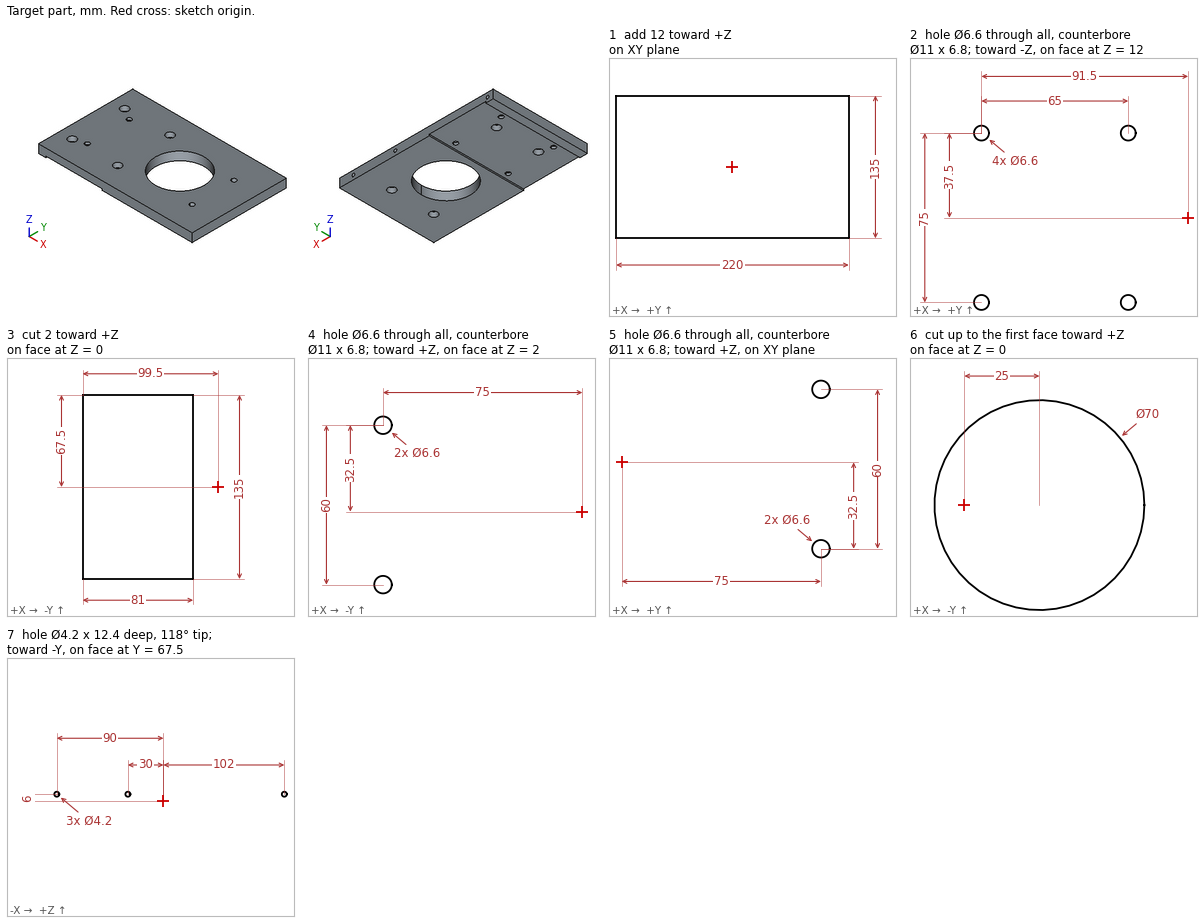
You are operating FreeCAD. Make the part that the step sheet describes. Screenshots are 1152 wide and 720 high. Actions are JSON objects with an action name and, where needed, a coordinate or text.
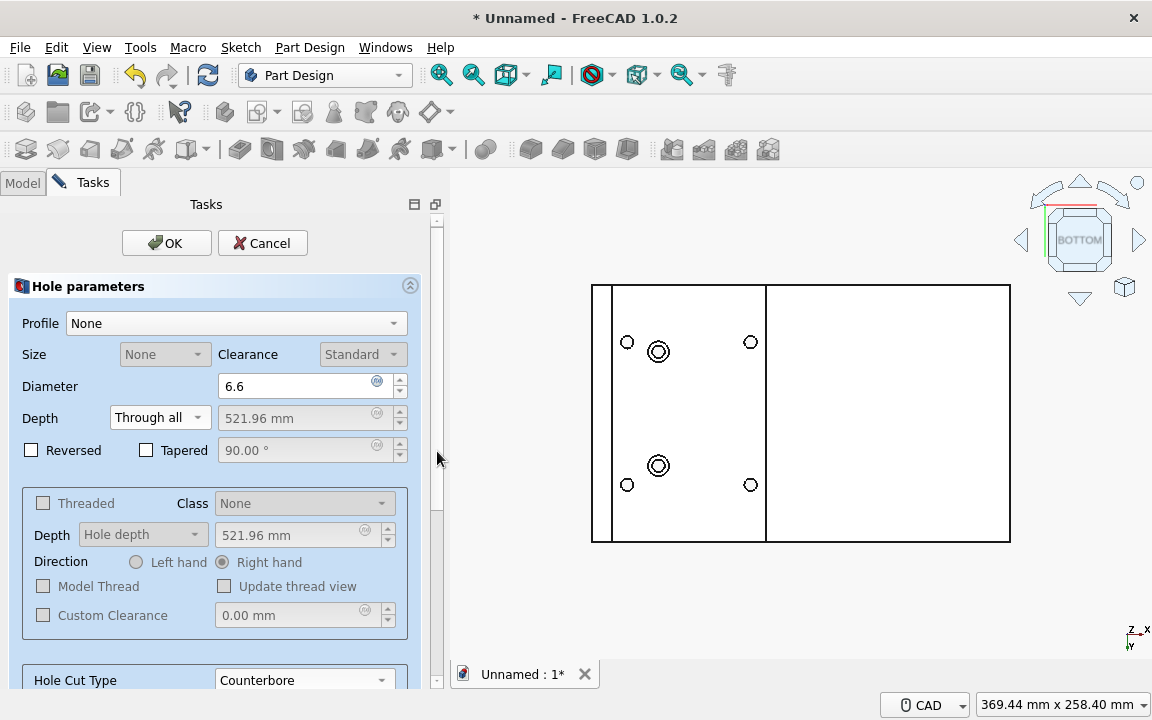
{"action": "left_click", "coordinate": [167, 243]}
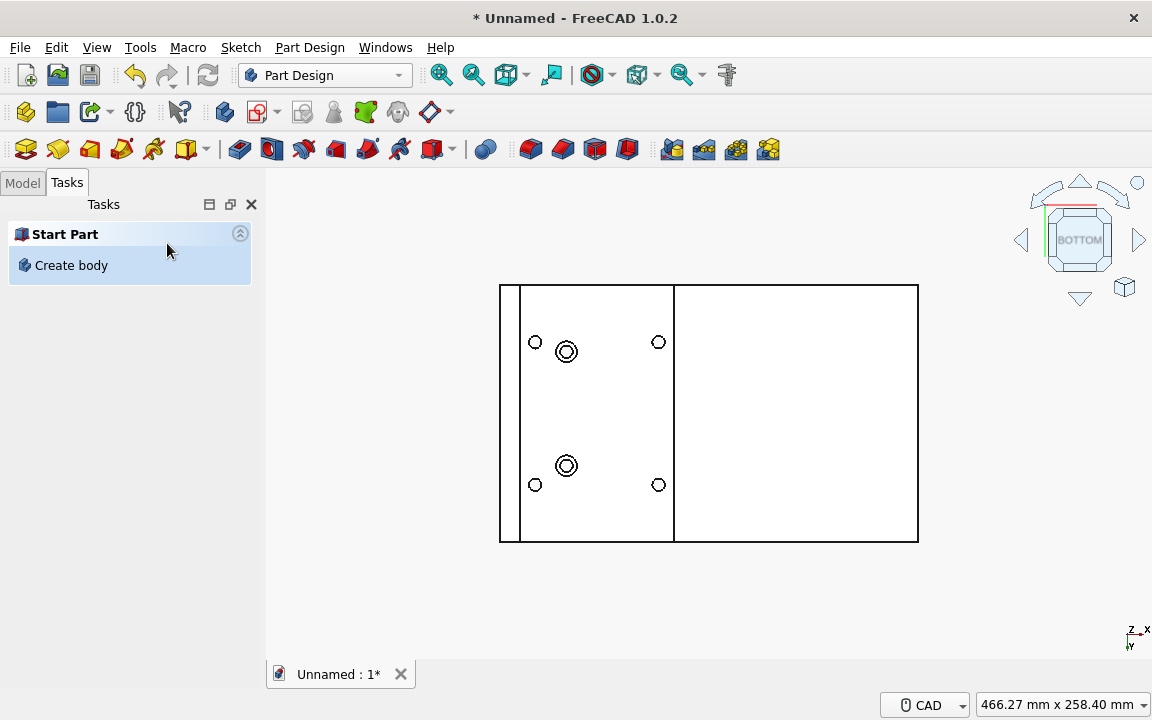
{"action": "left_click", "coordinate": [258, 112]}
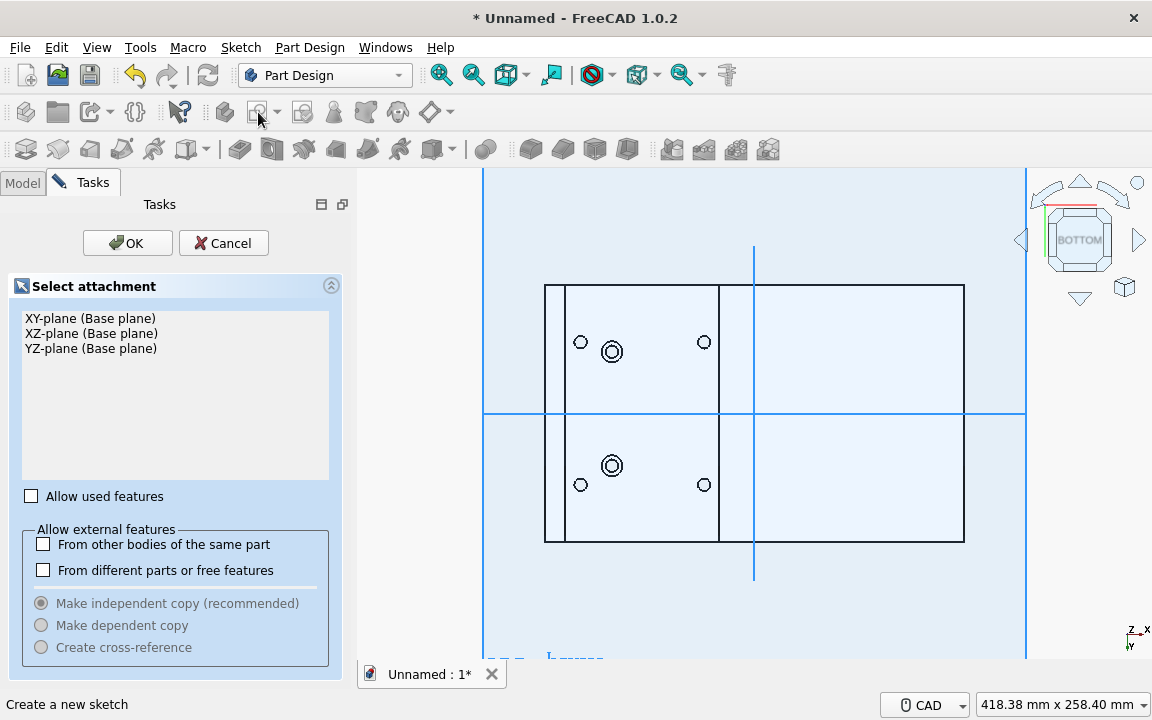
{"action": "left_click", "coordinate": [82, 318]}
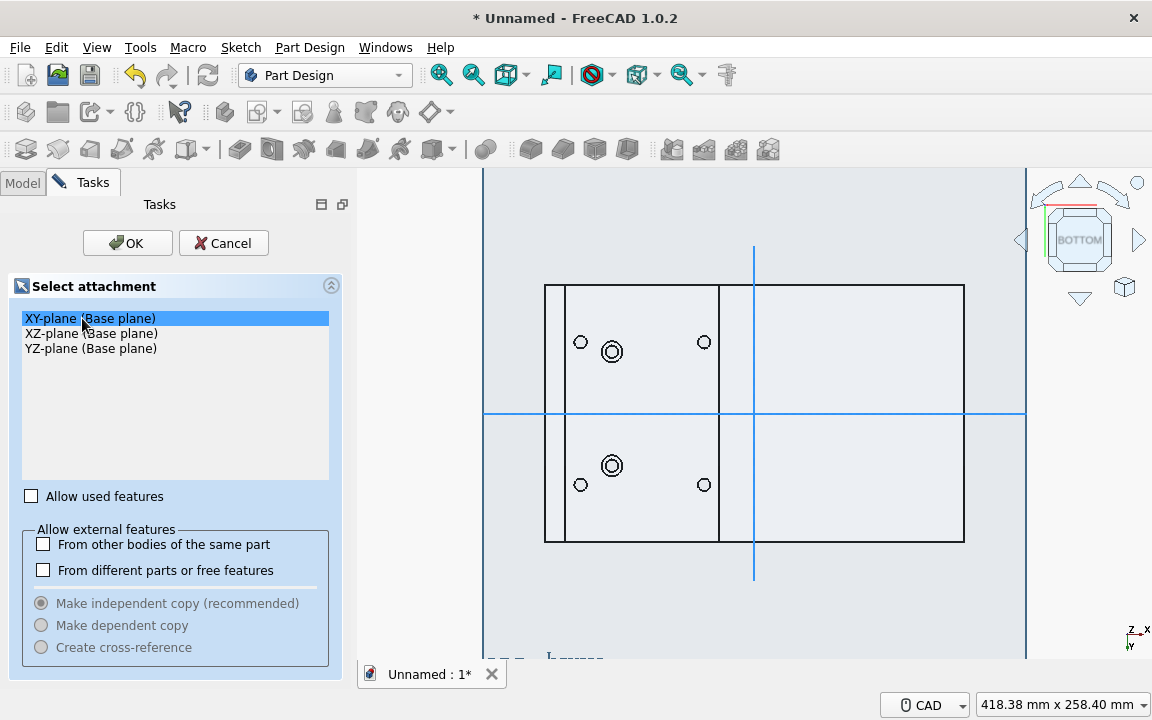
{"action": "left_click", "coordinate": [128, 243]}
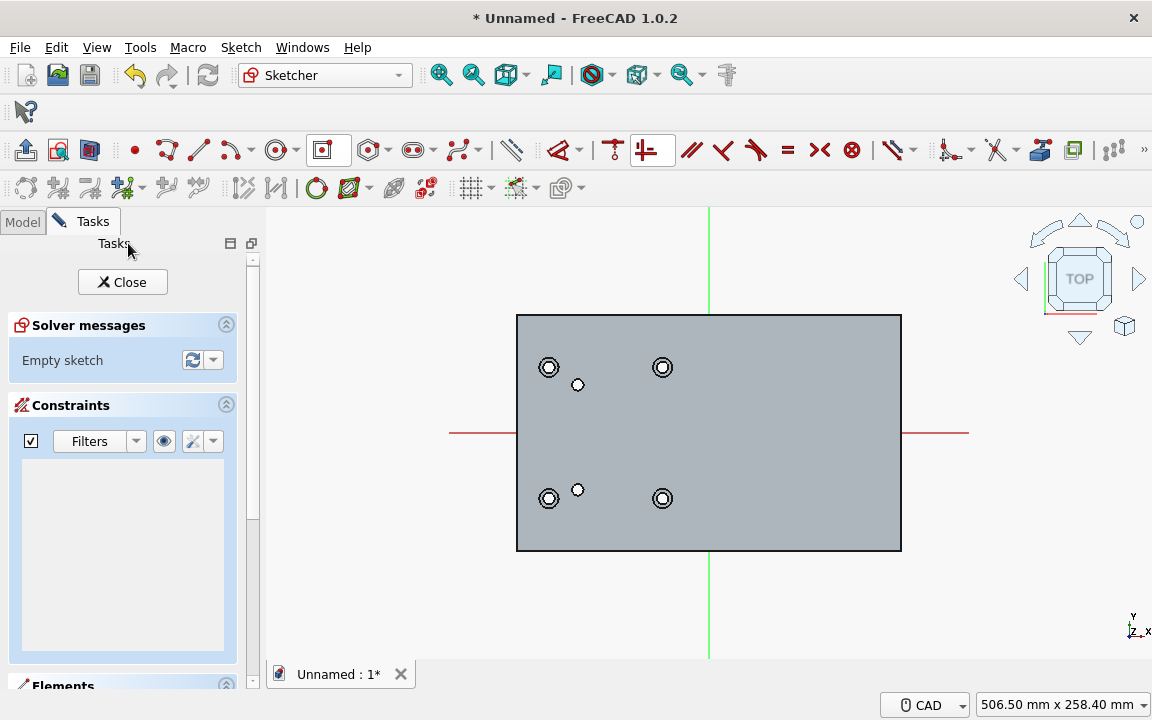
{"action": "key", "text": "q s"}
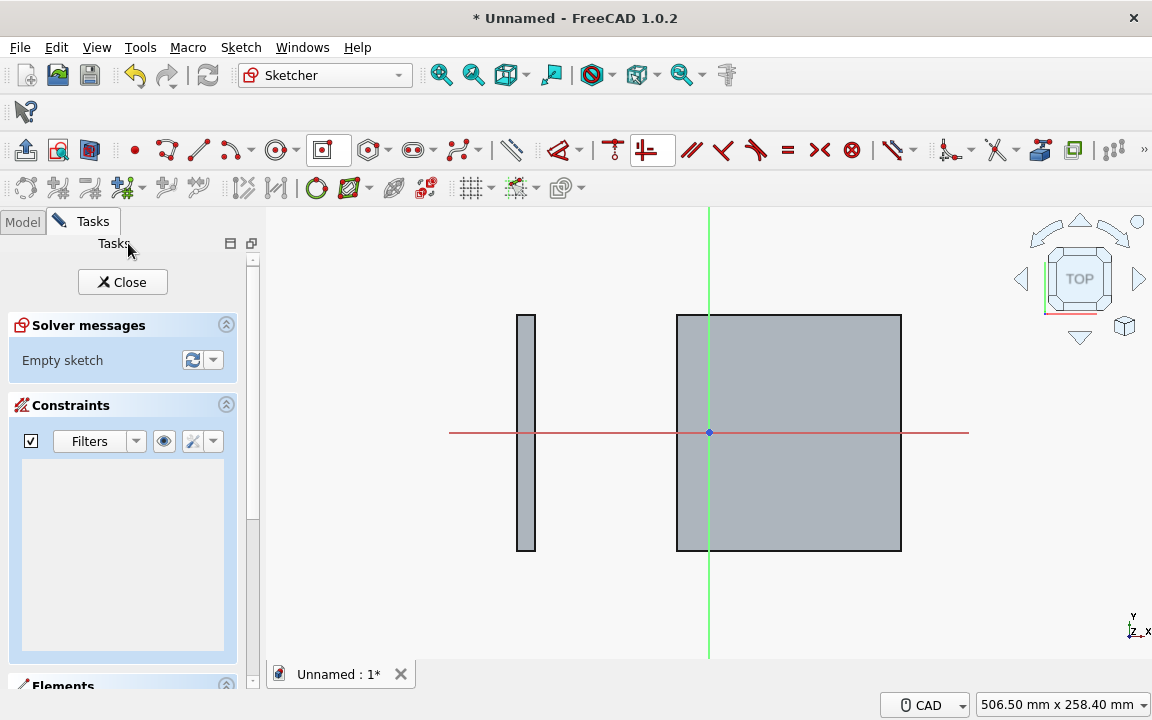
{"action": "scroll", "coordinate": [889, 441], "scroll_direction": "up", "scroll_amount": 4}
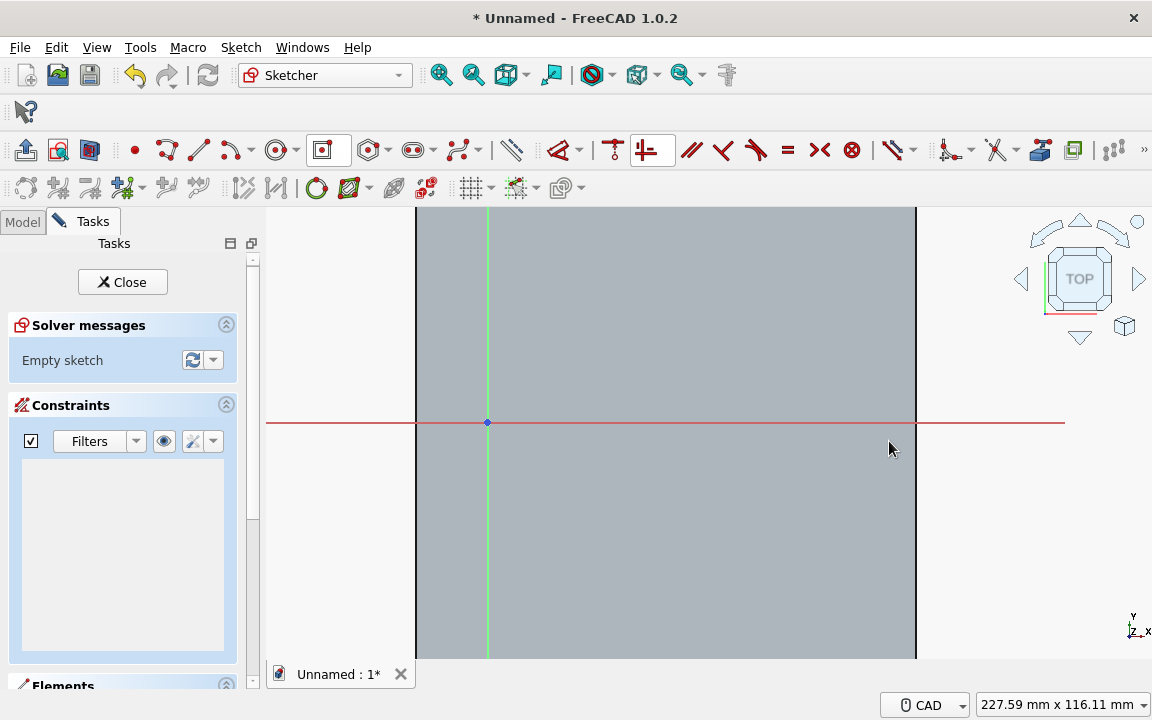
{"action": "key", "text": "g c"}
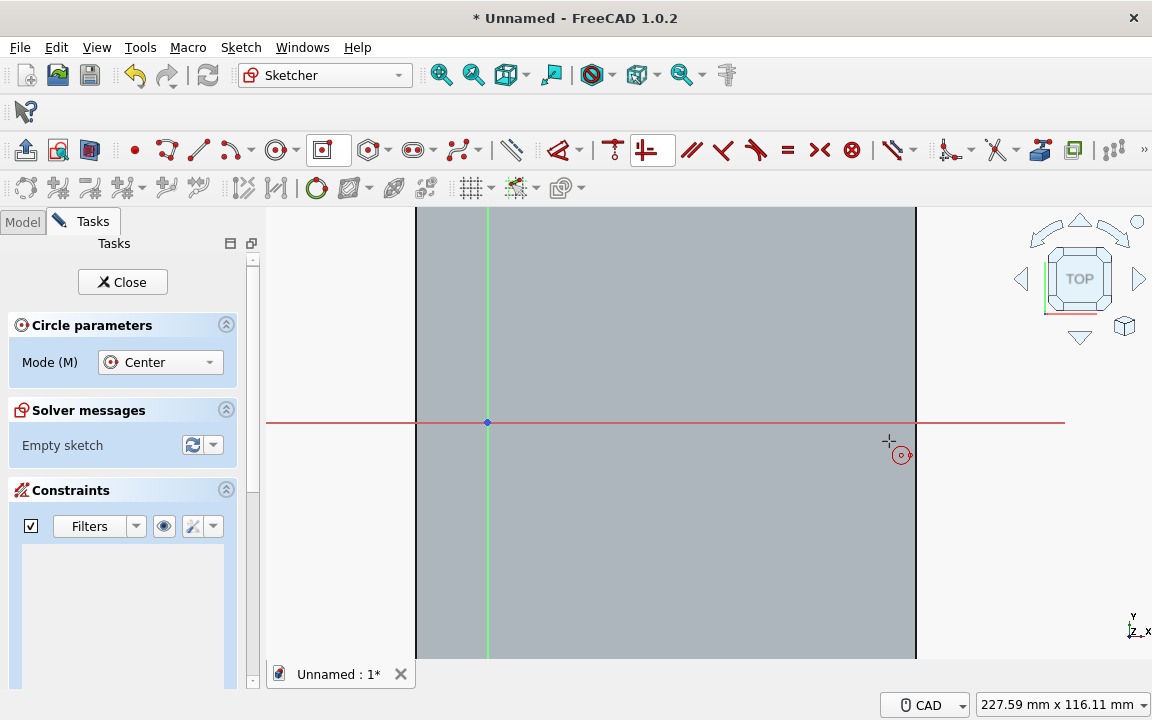
{"action": "scroll", "coordinate": [780, 549], "scroll_direction": "up", "scroll_amount": 3}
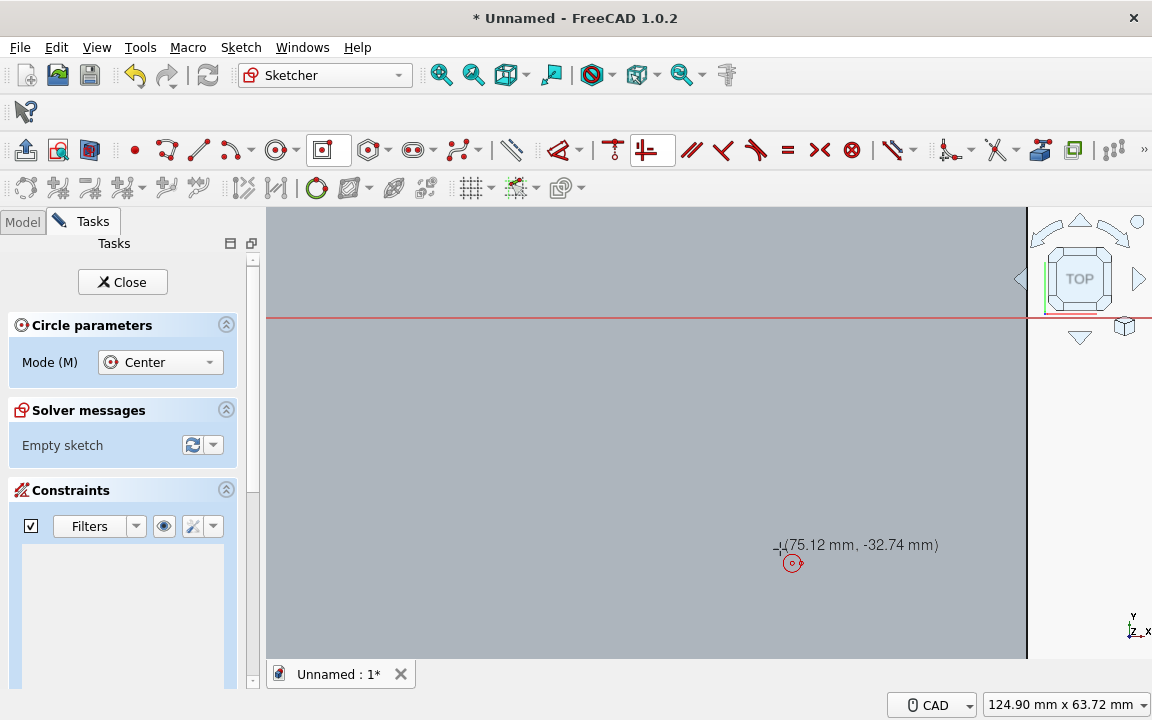
{"action": "left_click", "coordinate": [779, 549]}
{"action": "mouse_move", "coordinate": [795, 532]}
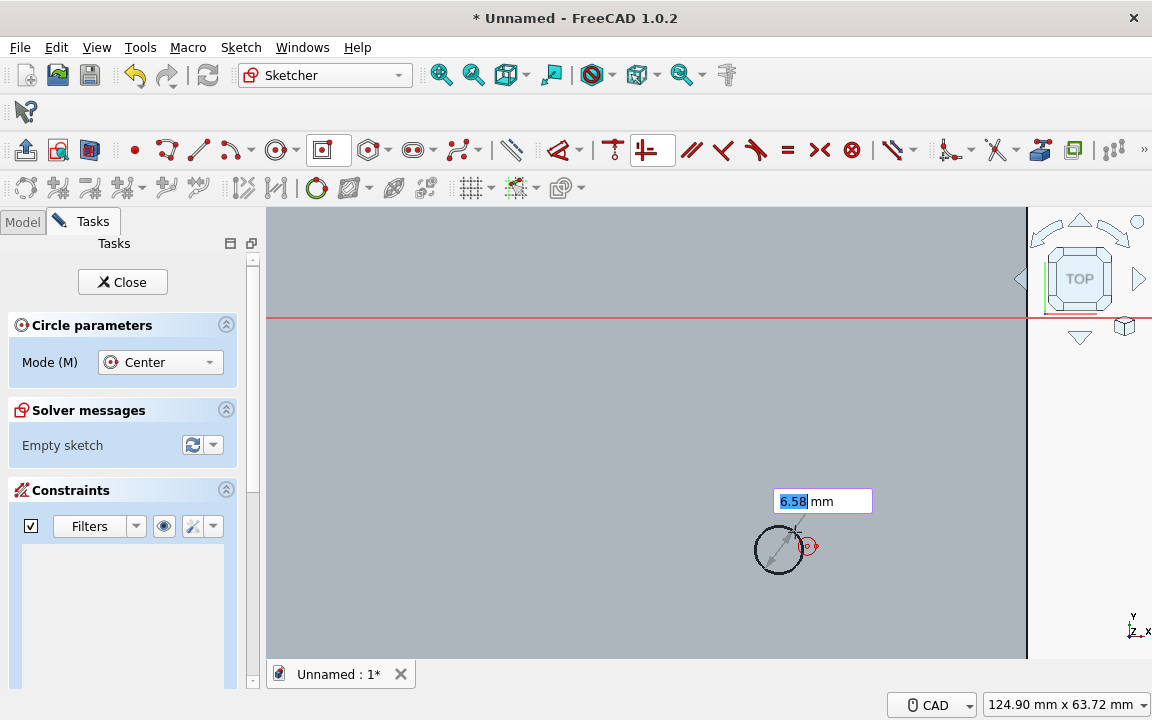
{"action": "type", "text": "6.6"}
{"action": "key", "text": "Return"}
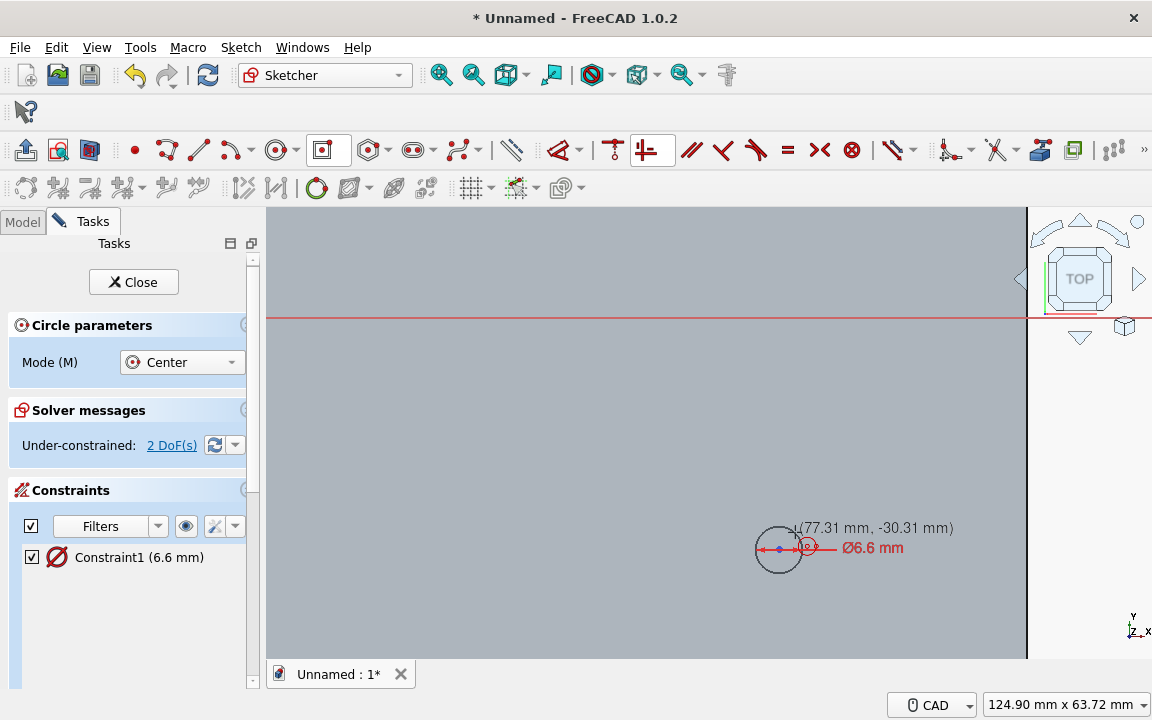
{"action": "scroll", "coordinate": [782, 551], "scroll_direction": "down", "scroll_amount": 3}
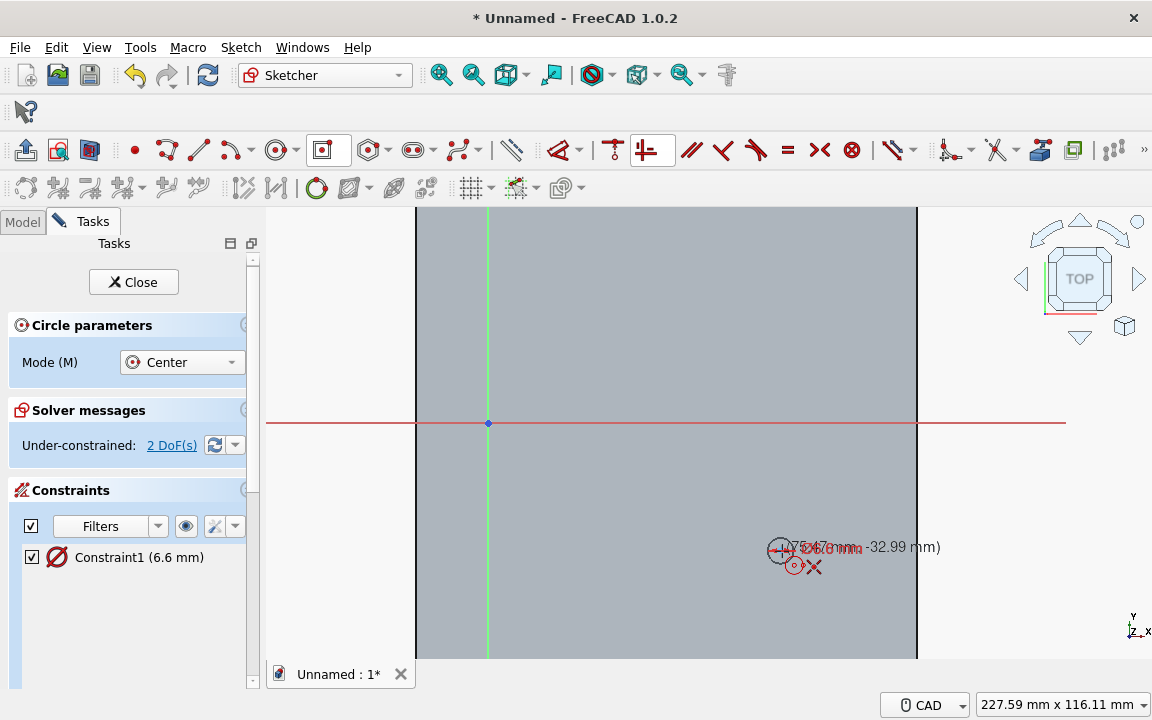
{"action": "scroll", "coordinate": [780, 316], "scroll_direction": "up", "scroll_amount": 3}